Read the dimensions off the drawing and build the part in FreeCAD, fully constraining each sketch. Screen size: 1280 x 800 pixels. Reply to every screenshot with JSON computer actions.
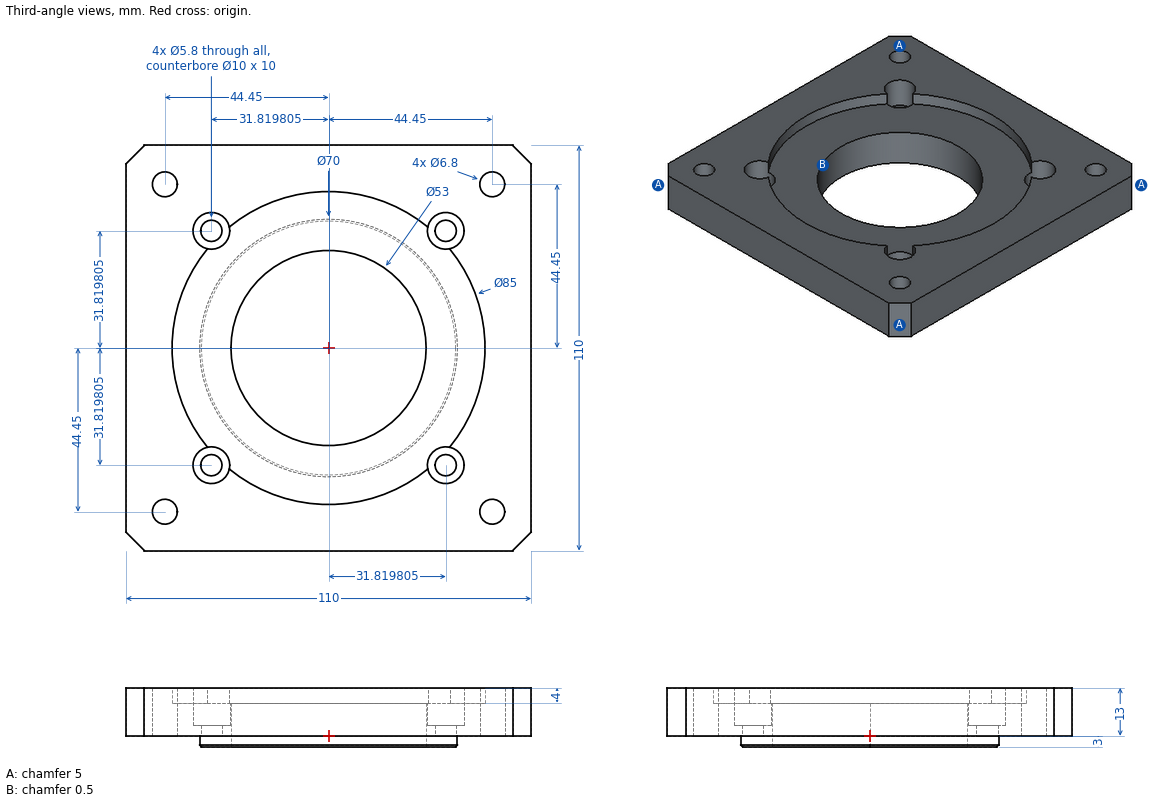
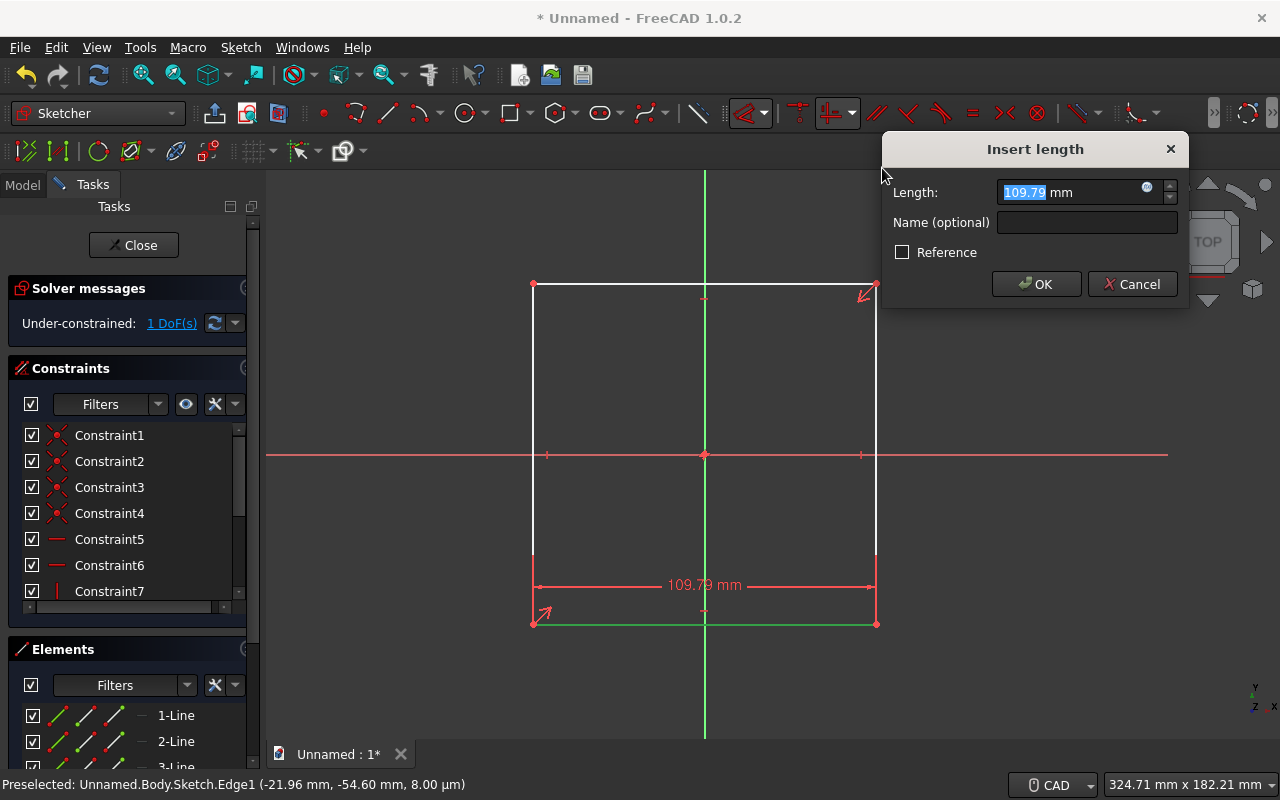
{"action": "type", "text": "110"}
{"action": "key", "text": "Return"}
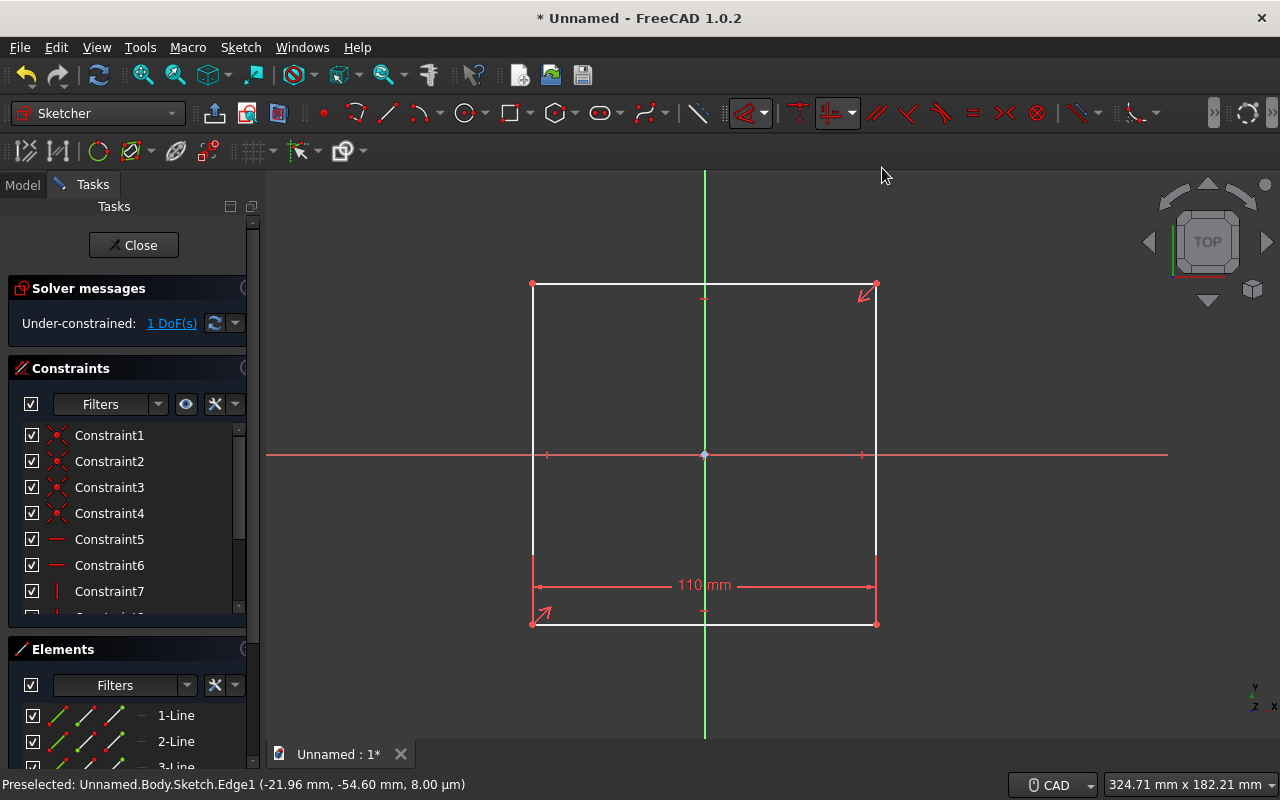
{"action": "left_click", "coordinate": [876, 523]}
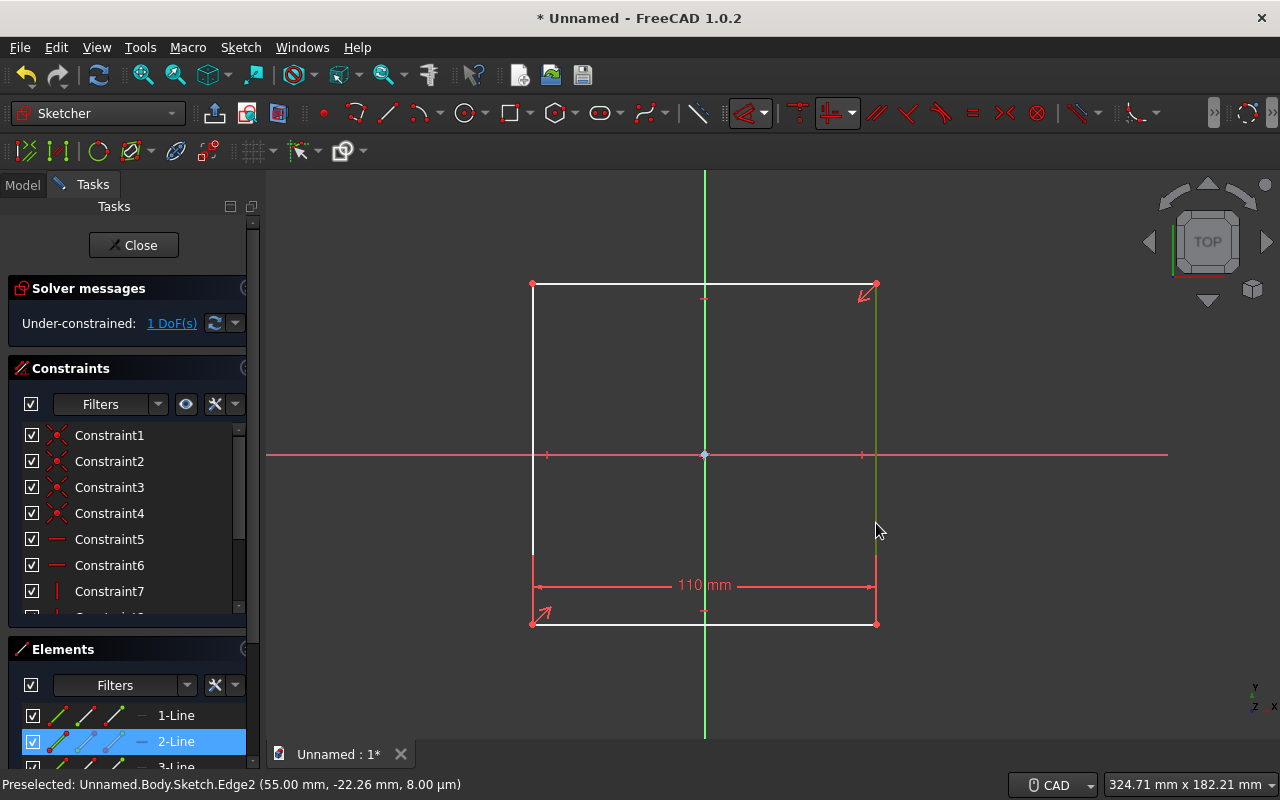
{"action": "left_click", "coordinate": [766, 114]}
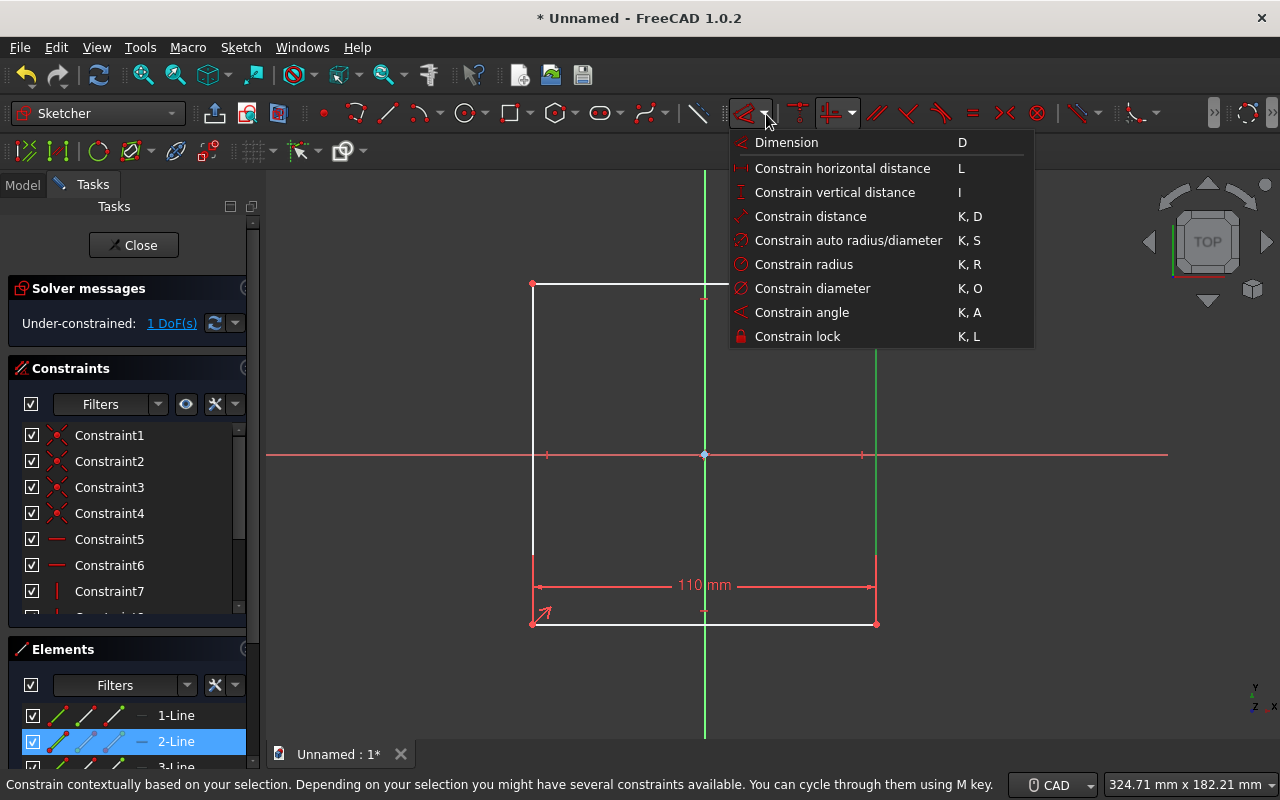
{"action": "left_click", "coordinate": [882, 192]}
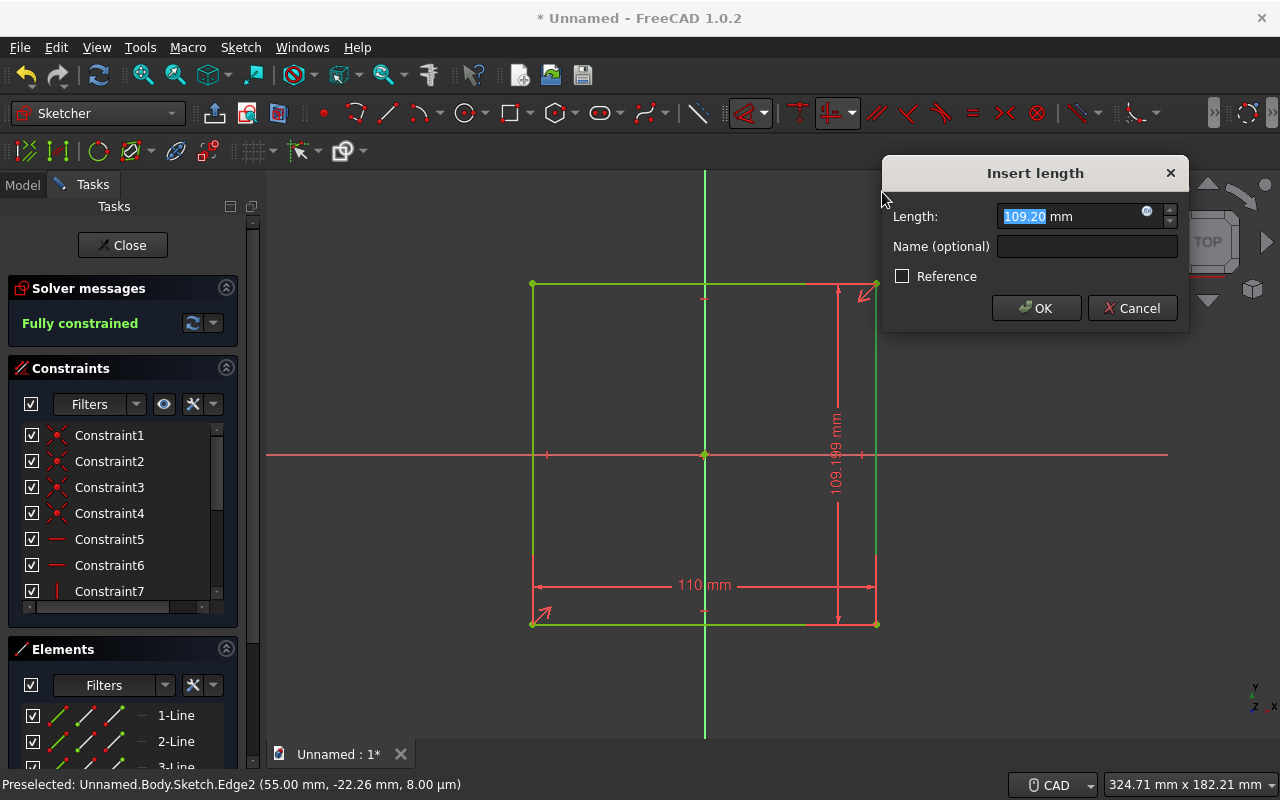
{"action": "type", "text": "110"}
{"action": "key", "text": "Return"}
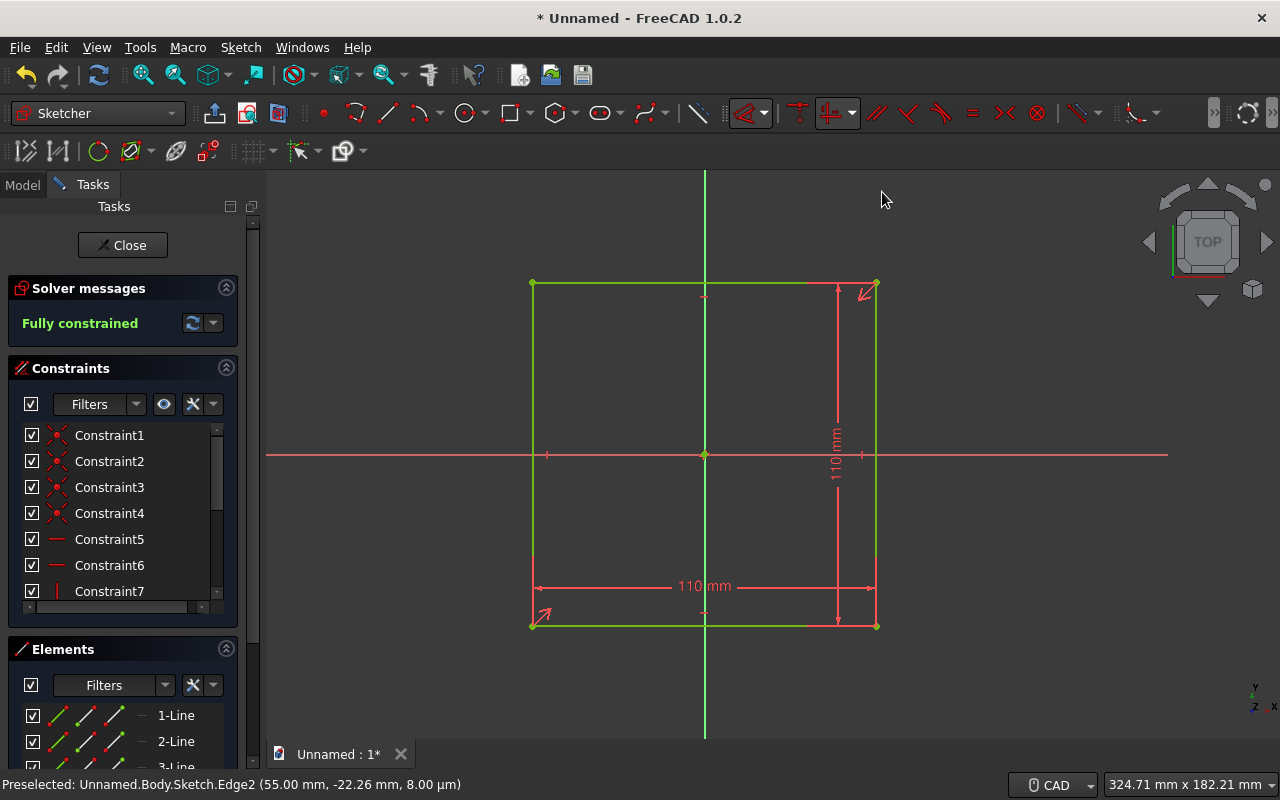
{"action": "left_click", "coordinate": [123, 245]}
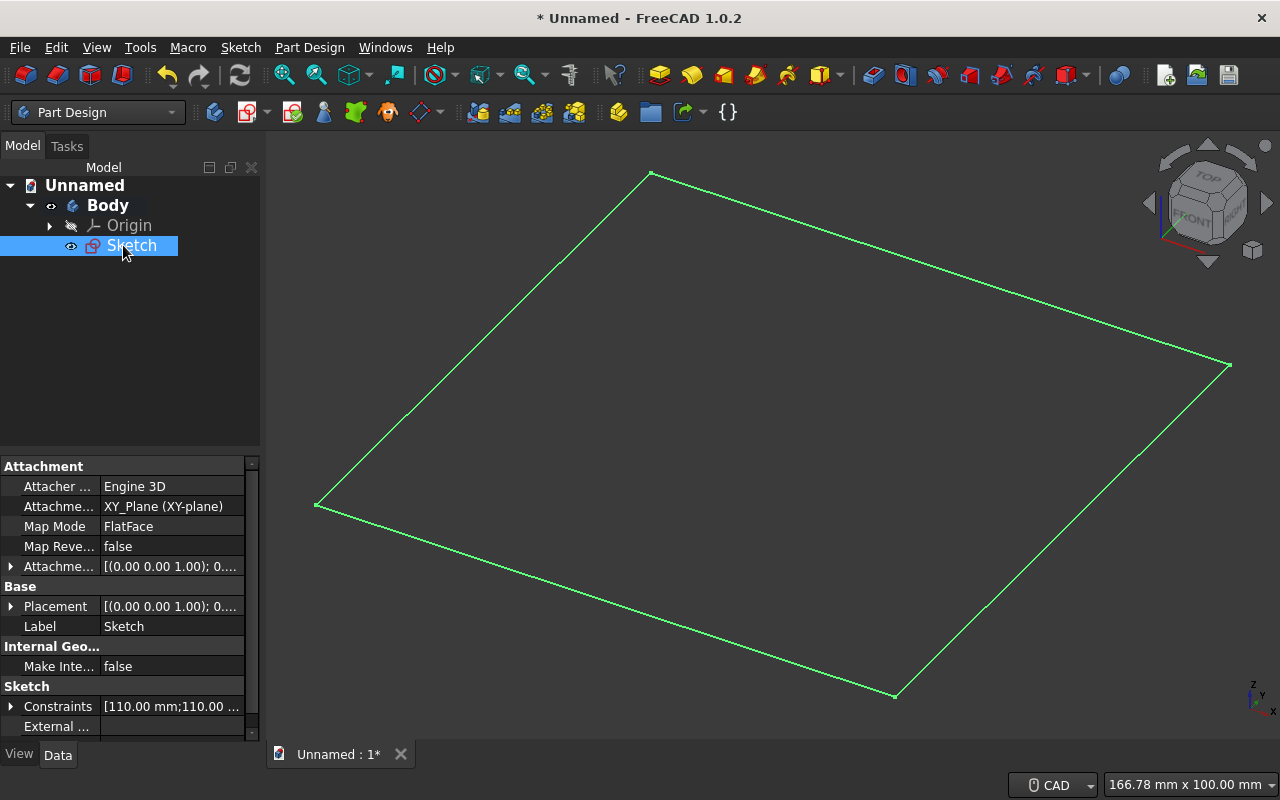
{"action": "left_click", "coordinate": [660, 76]}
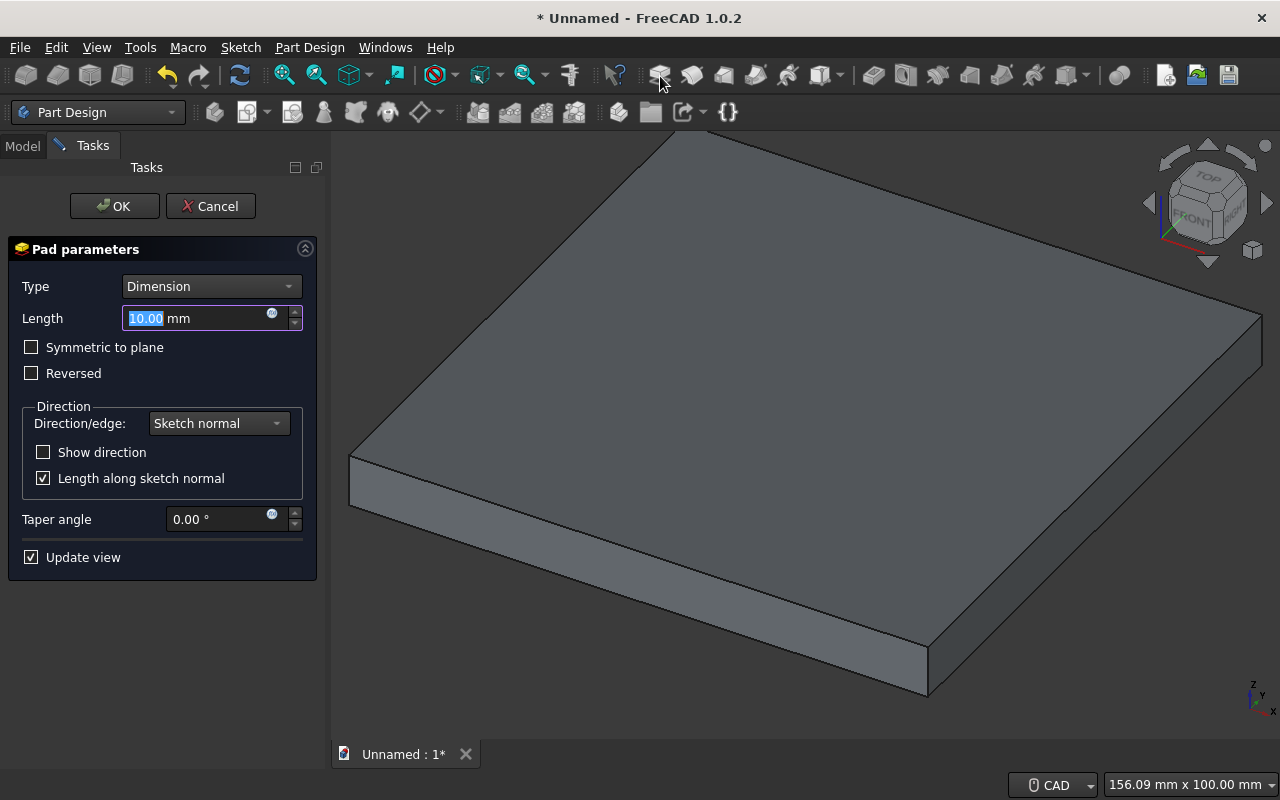
{"action": "type", "text": "13"}
{"action": "key", "text": "Tab"}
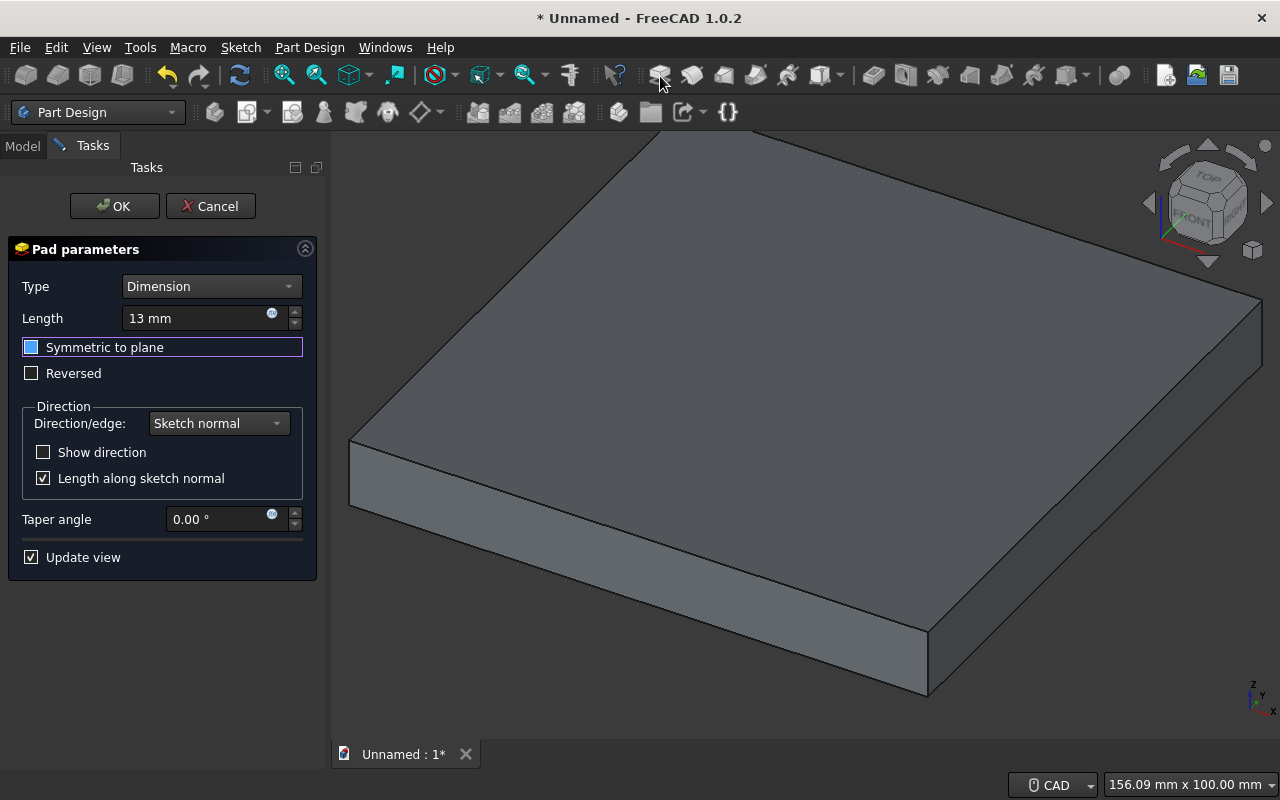
{"action": "left_click", "coordinate": [115, 206]}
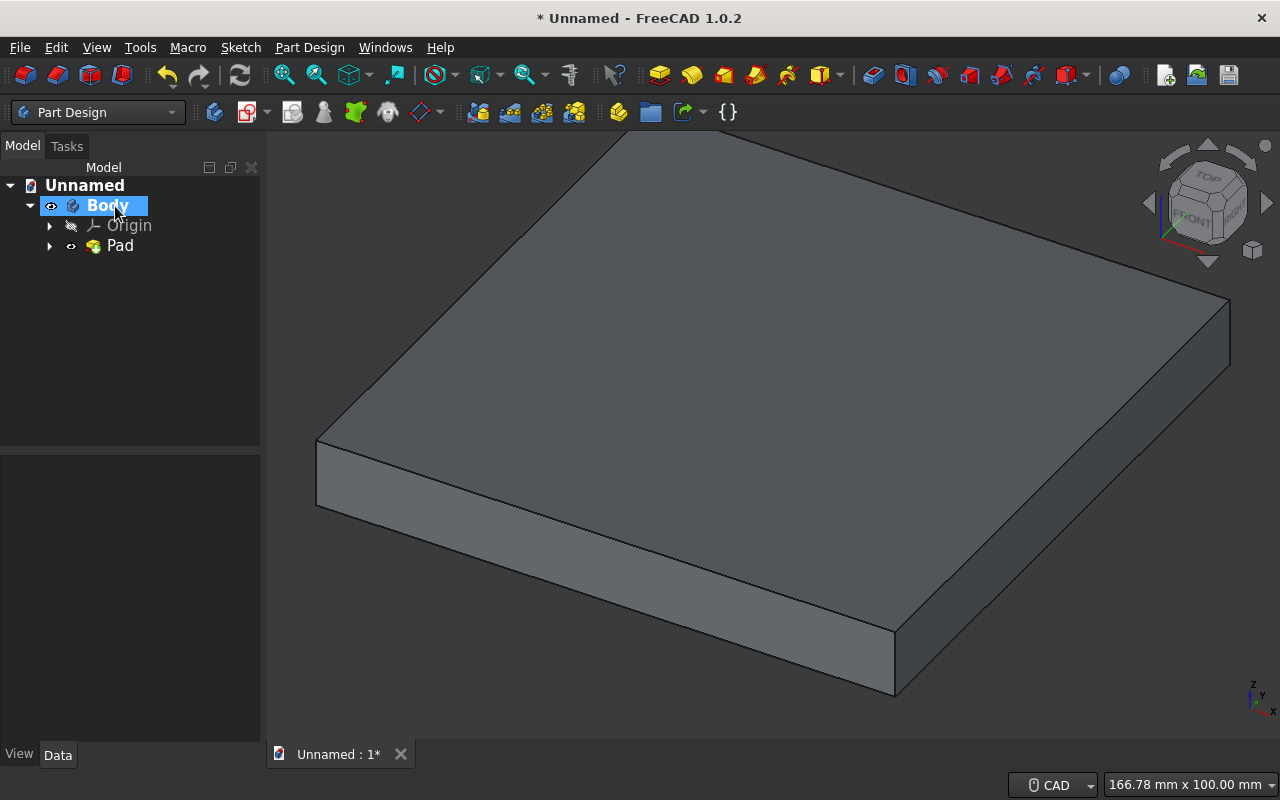
{"action": "left_click", "coordinate": [286, 76]}